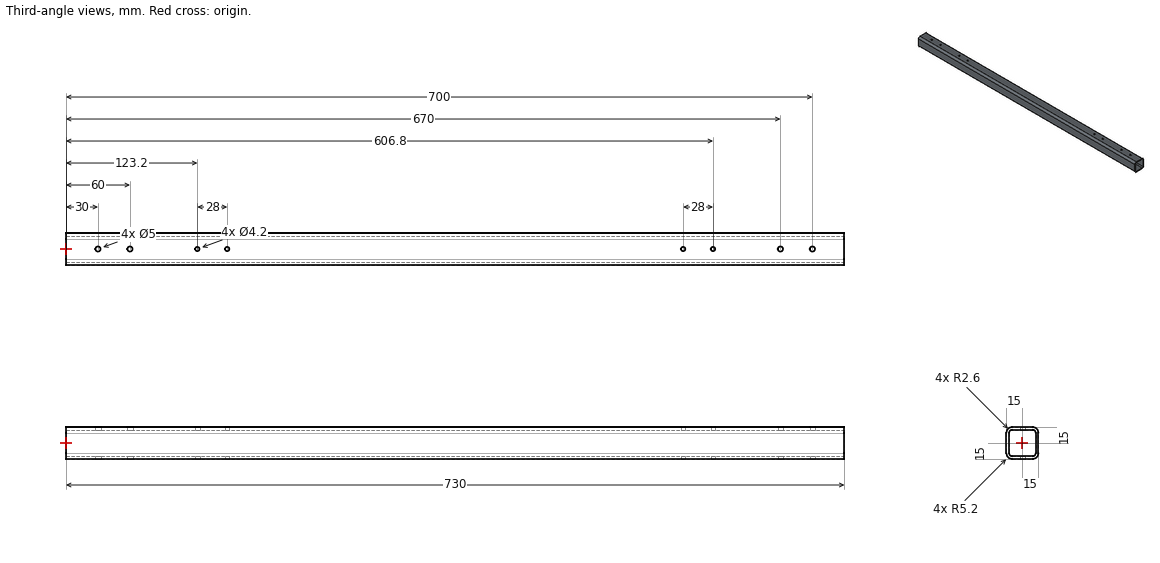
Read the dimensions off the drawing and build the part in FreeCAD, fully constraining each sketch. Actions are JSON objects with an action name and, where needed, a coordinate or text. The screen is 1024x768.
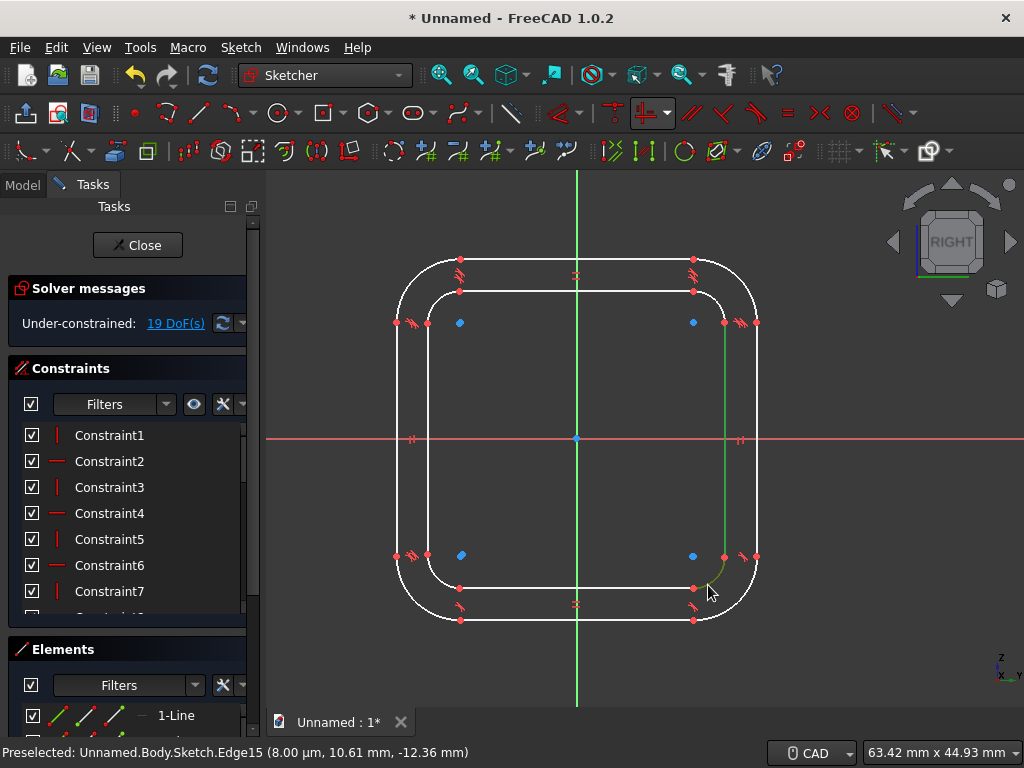
{"action": "left_click", "coordinate": [756, 114]}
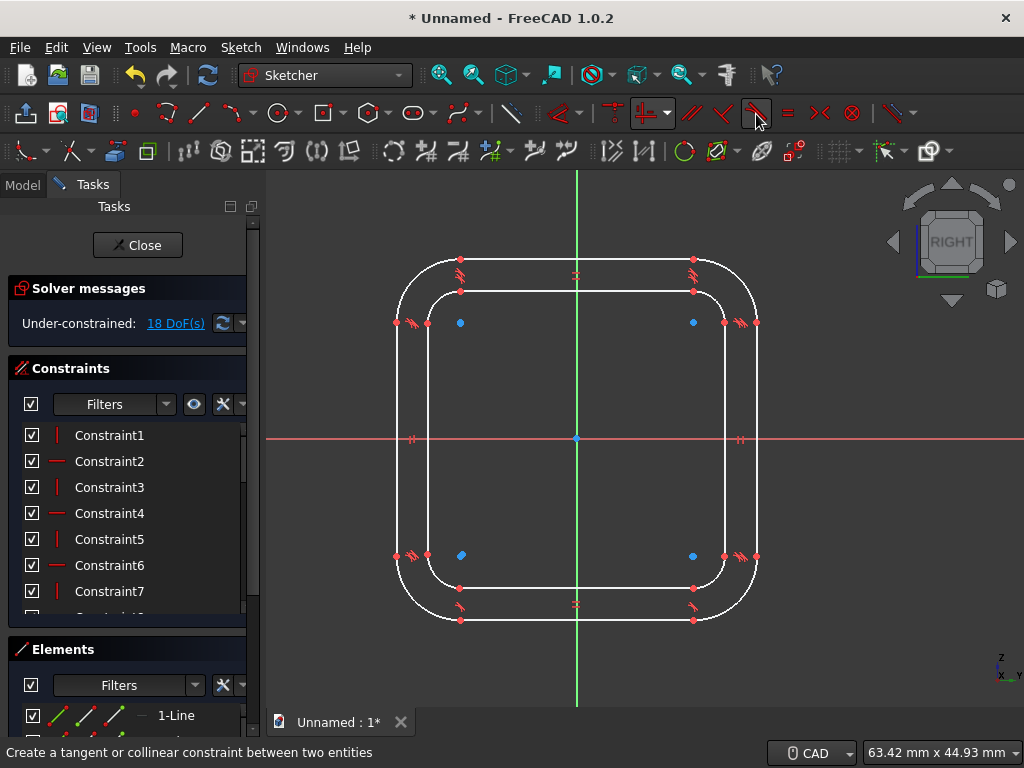
{"action": "left_click", "coordinate": [624, 588]}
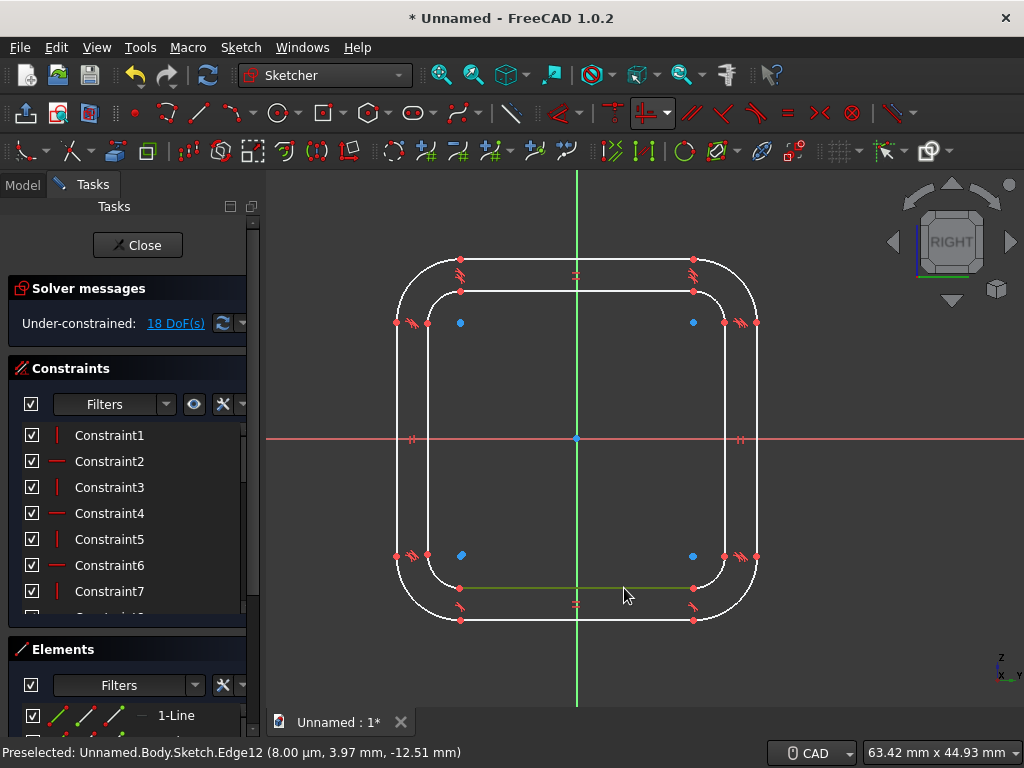
{"action": "left_click", "coordinate": [708, 585]}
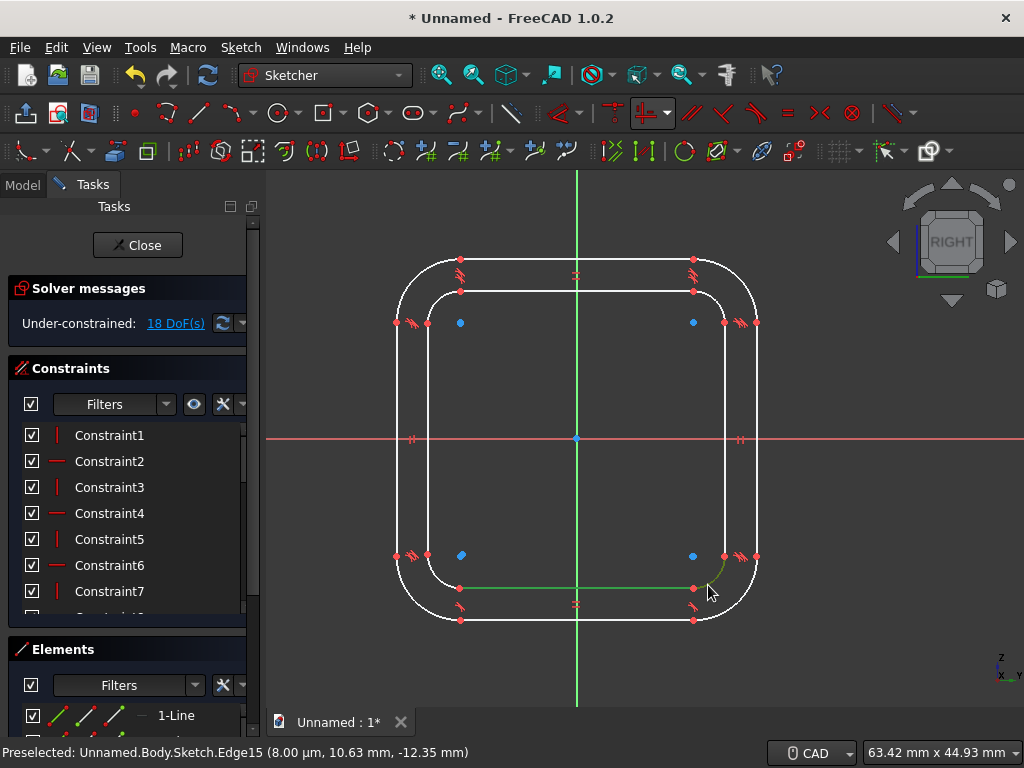
{"action": "left_click", "coordinate": [756, 114]}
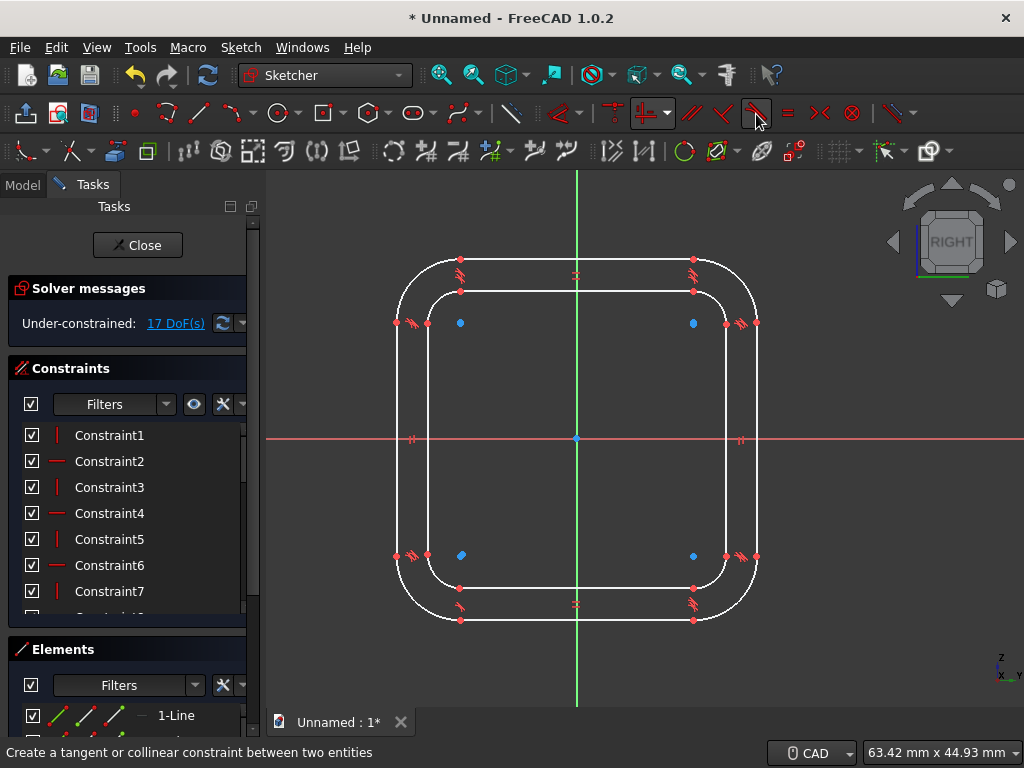
{"action": "left_click", "coordinate": [624, 588]}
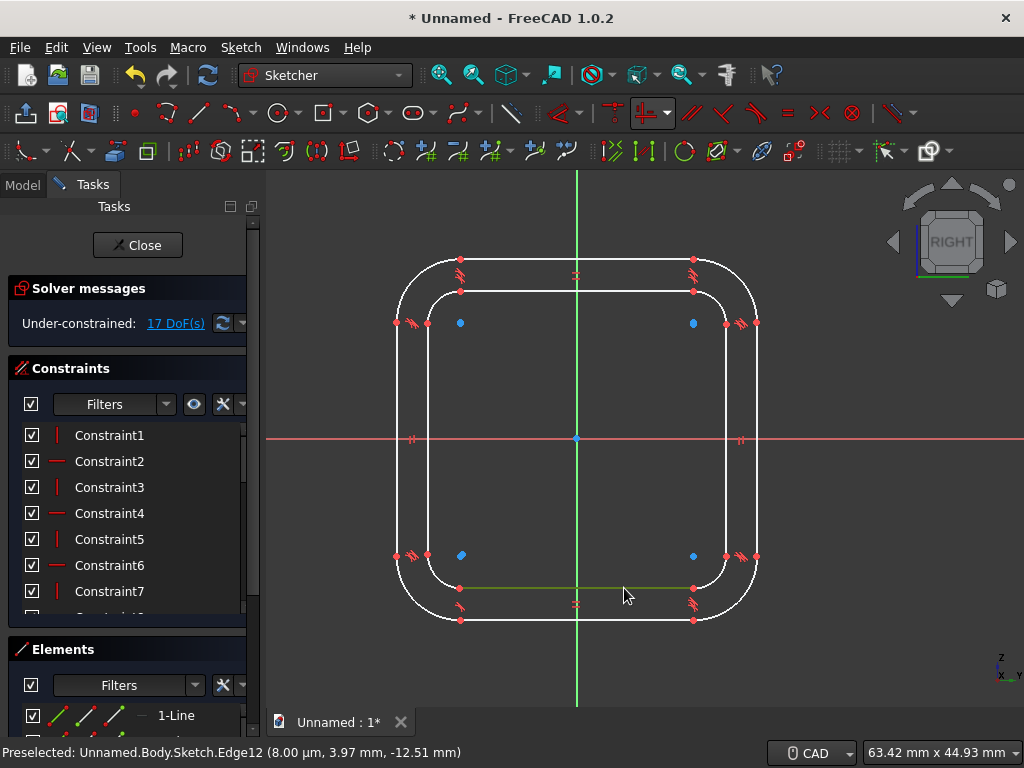
{"action": "left_click", "coordinate": [431, 569]}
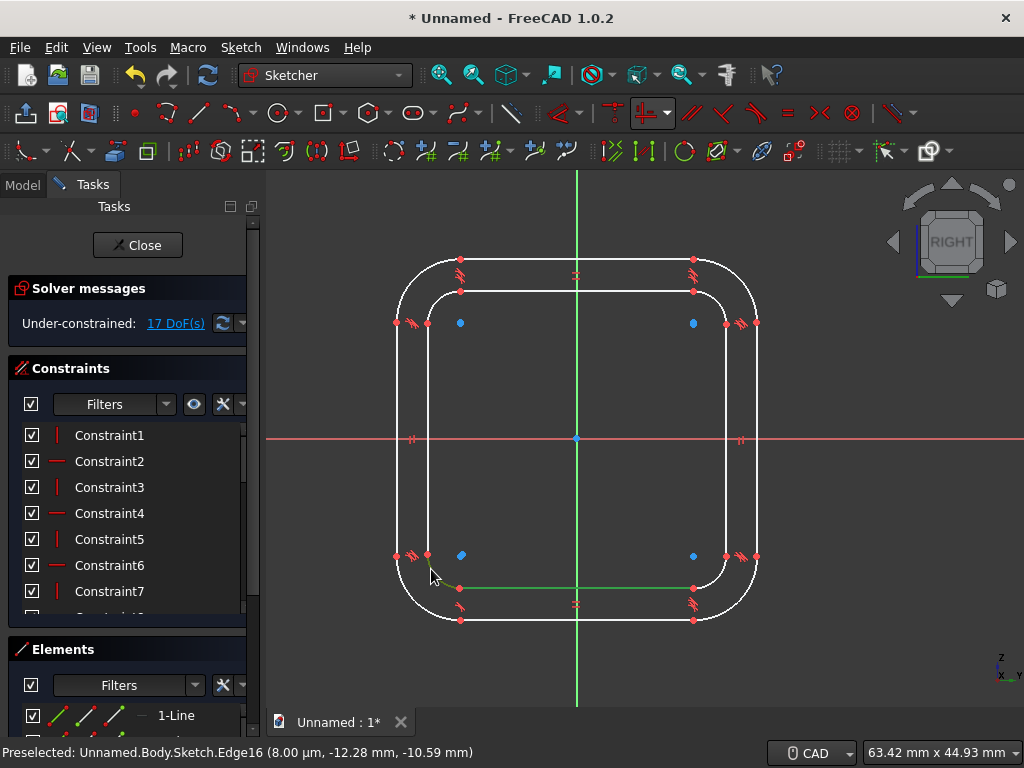
{"action": "left_click", "coordinate": [756, 114]}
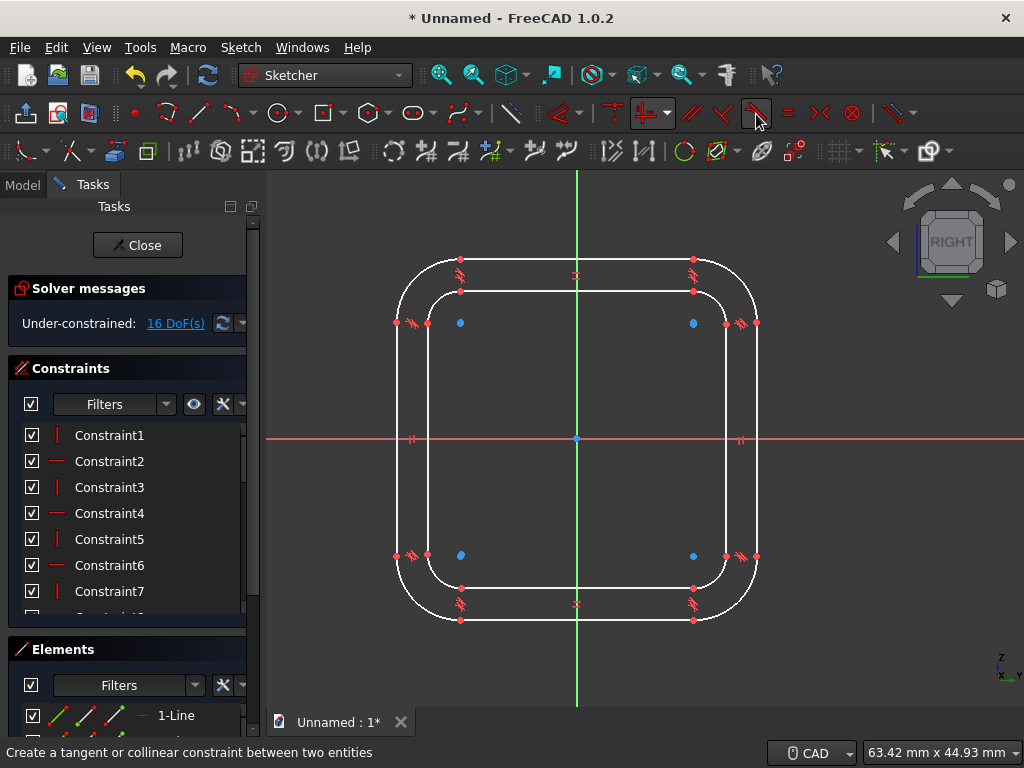
{"action": "left_click", "coordinate": [431, 266]}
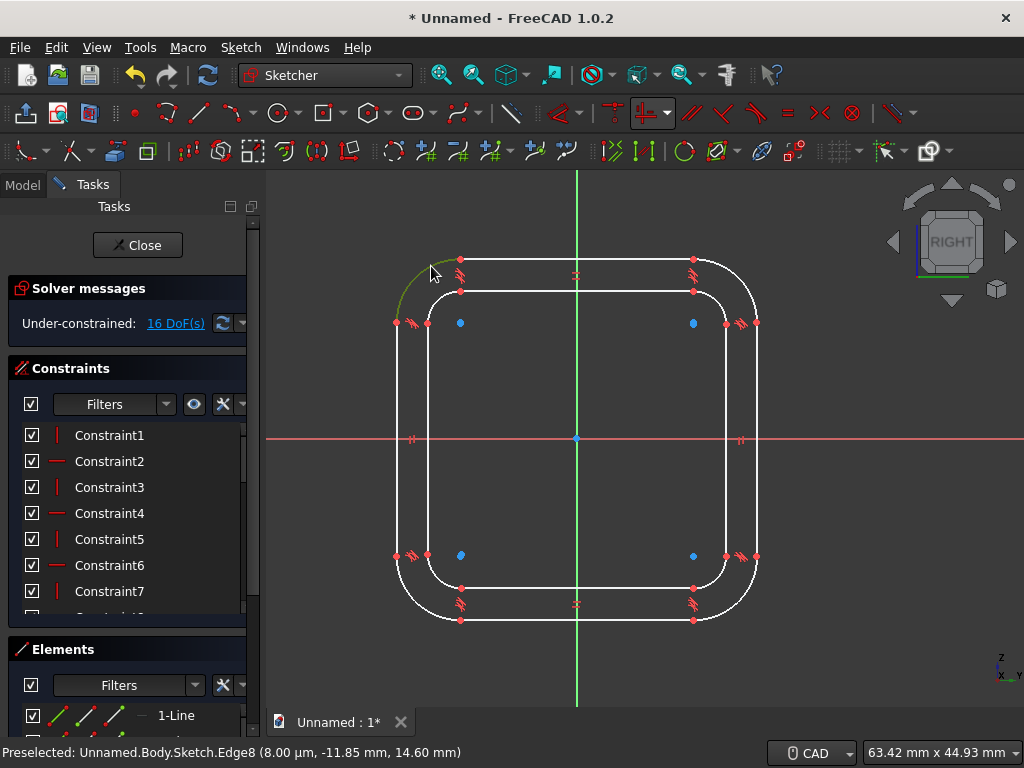
{"action": "left_click", "coordinate": [445, 295]}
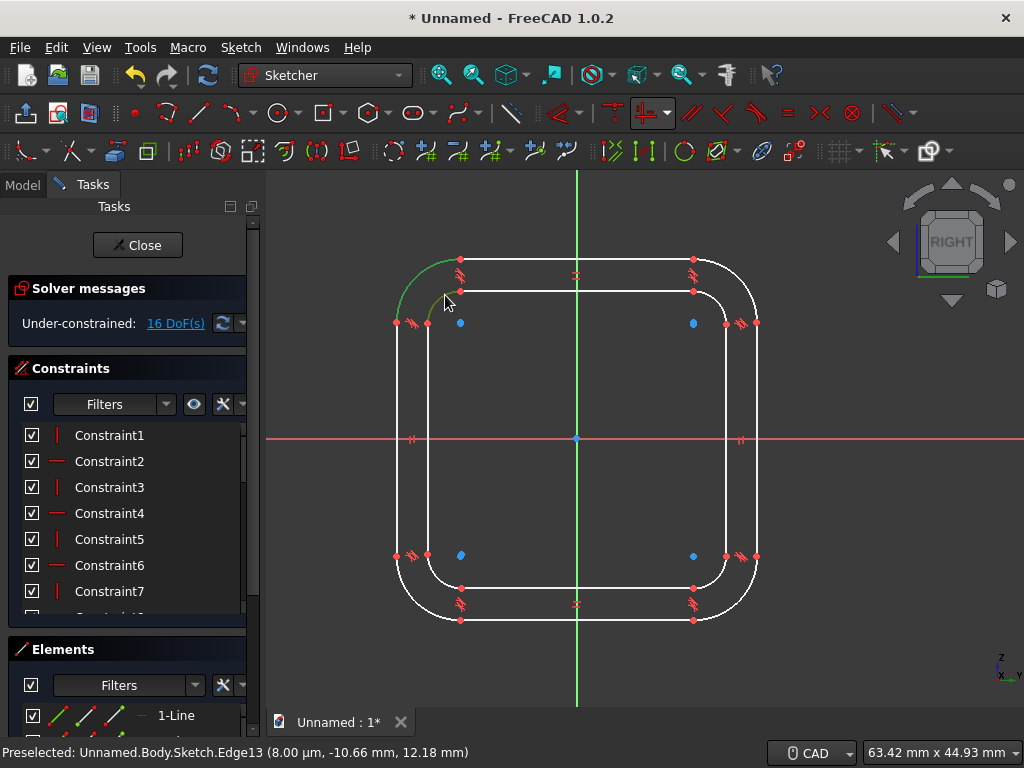
{"action": "left_click", "coordinate": [614, 114]}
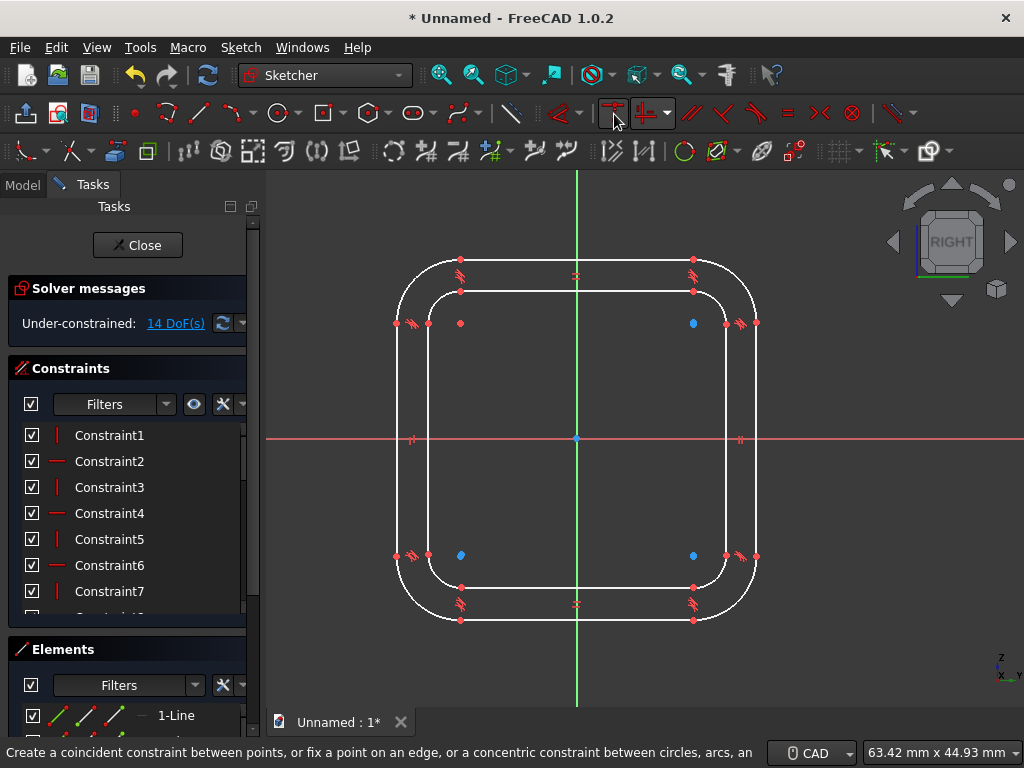
{"action": "left_click", "coordinate": [749, 294]}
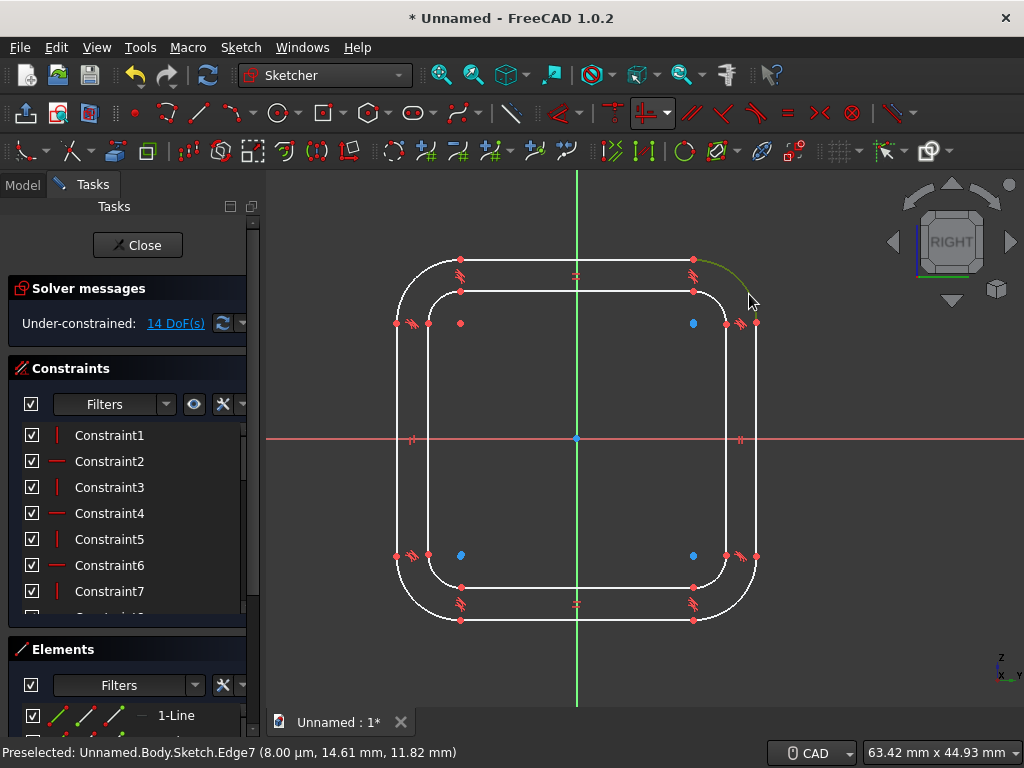
{"action": "left_click", "coordinate": [722, 309]}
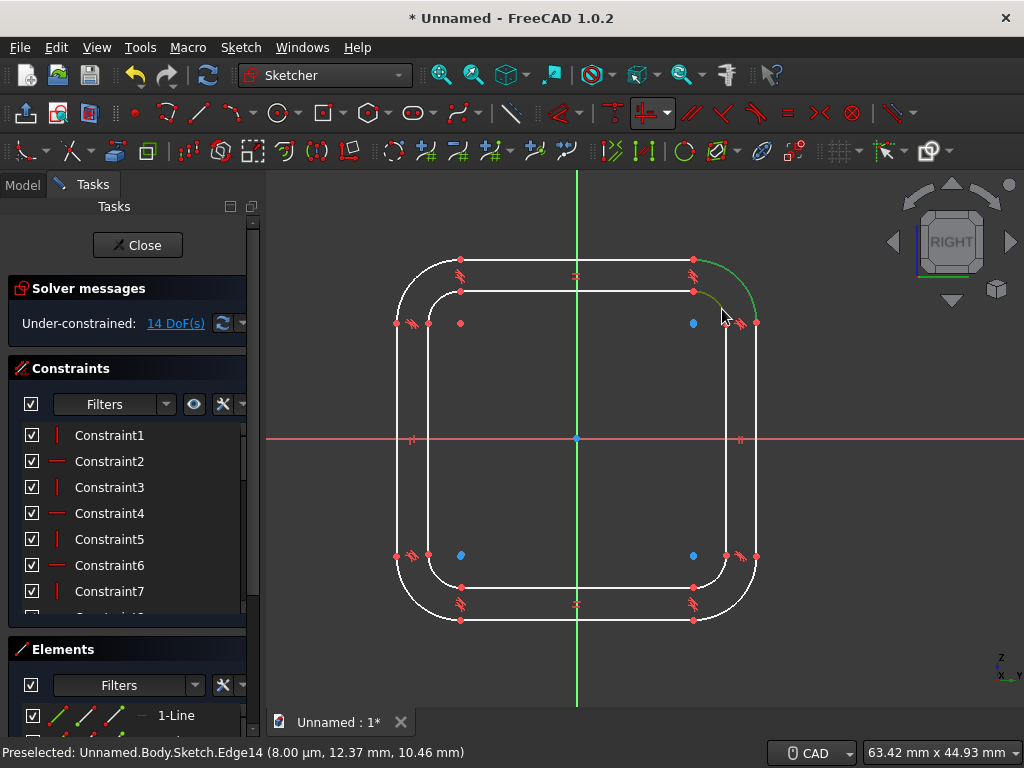
{"action": "left_click", "coordinate": [614, 114]}